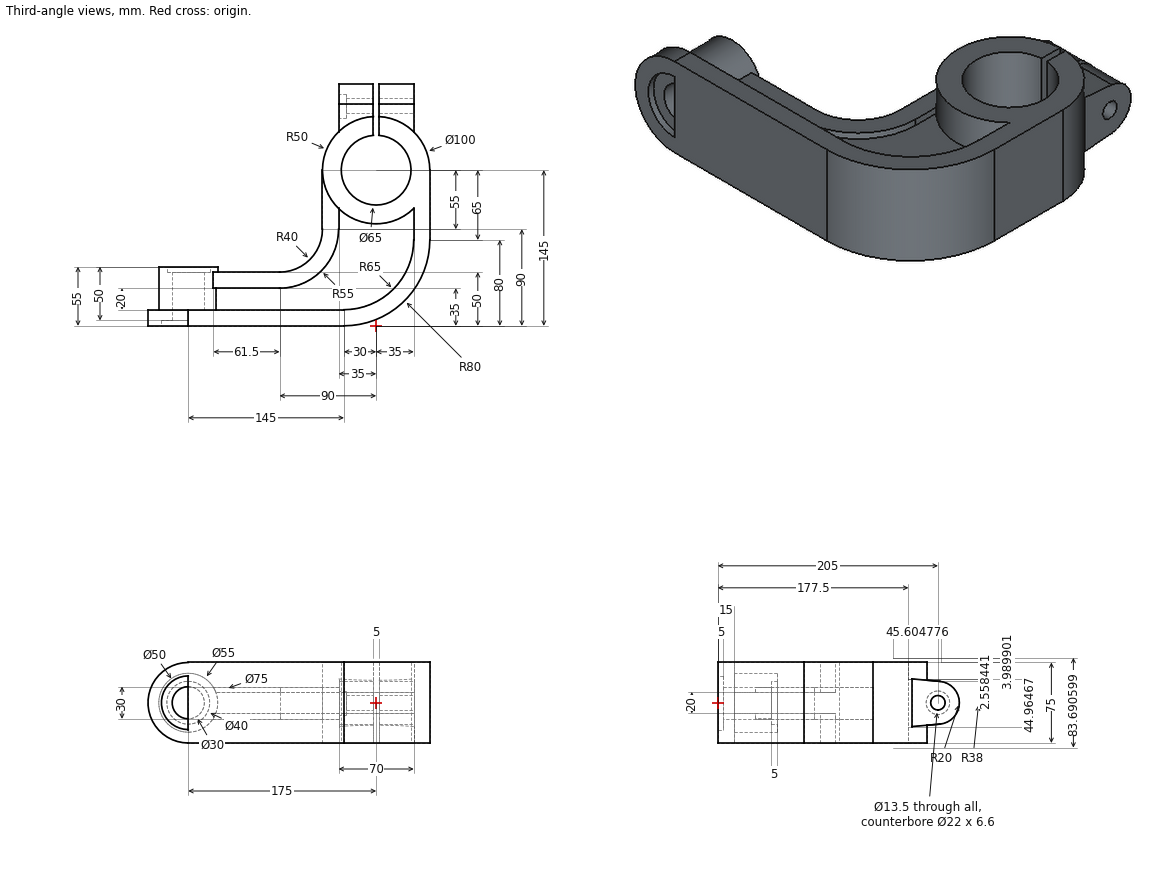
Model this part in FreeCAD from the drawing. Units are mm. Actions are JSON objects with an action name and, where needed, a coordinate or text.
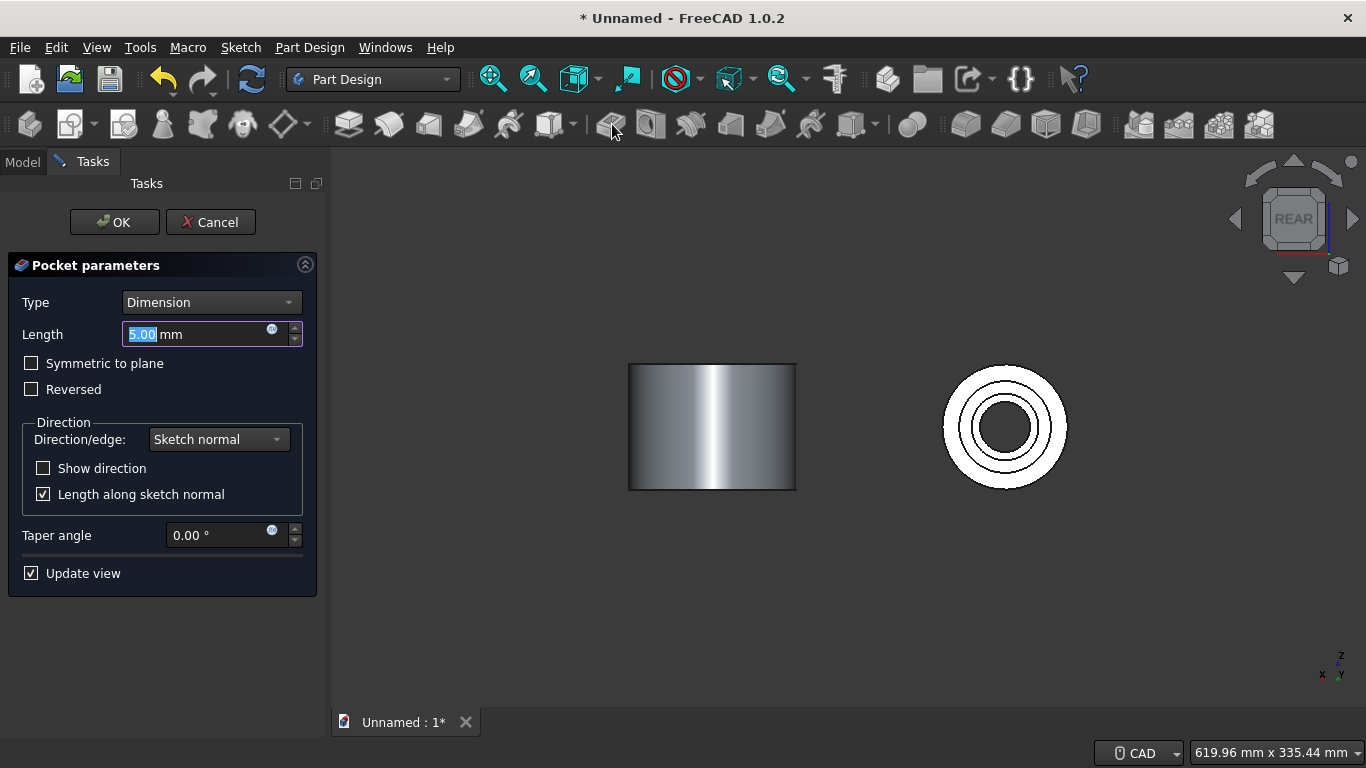
{"action": "type", "text": "5"}
{"action": "key", "text": "Tab"}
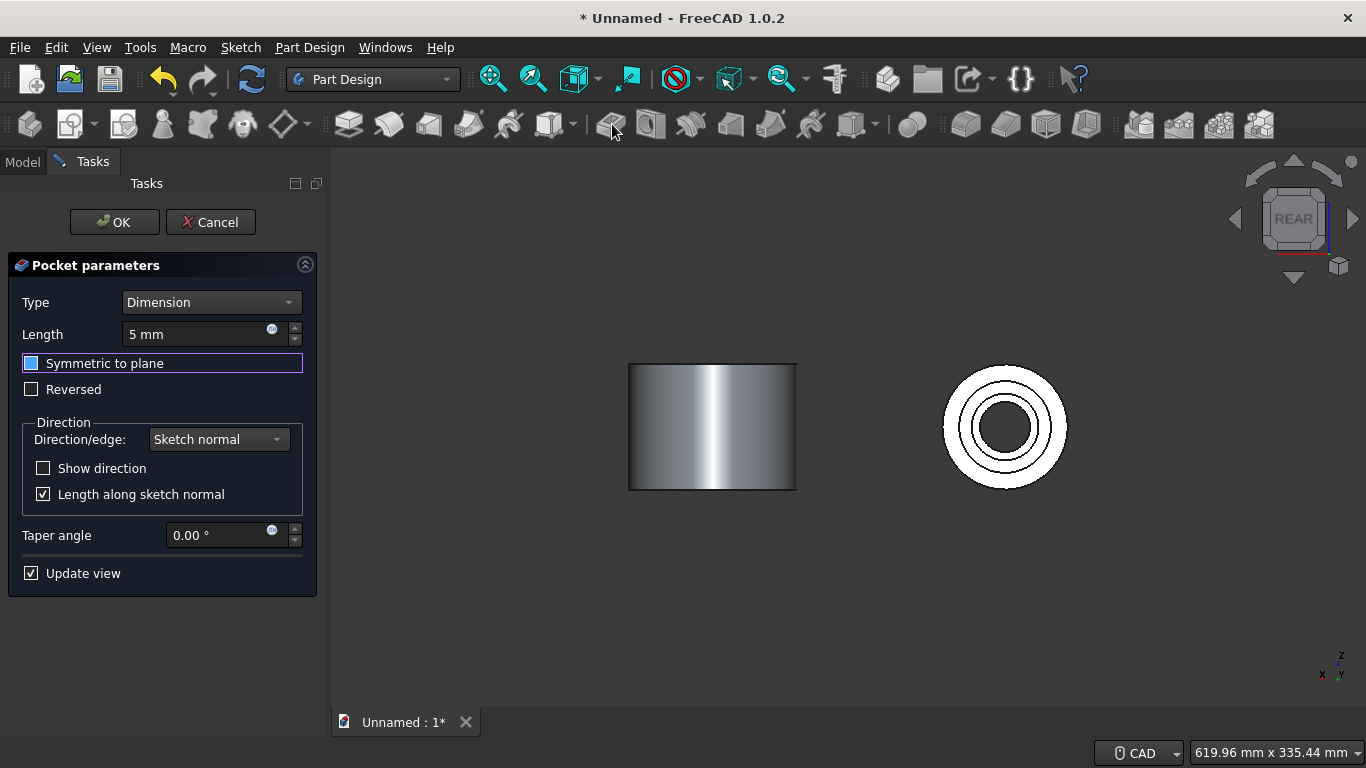
{"action": "left_click", "coordinate": [115, 222]}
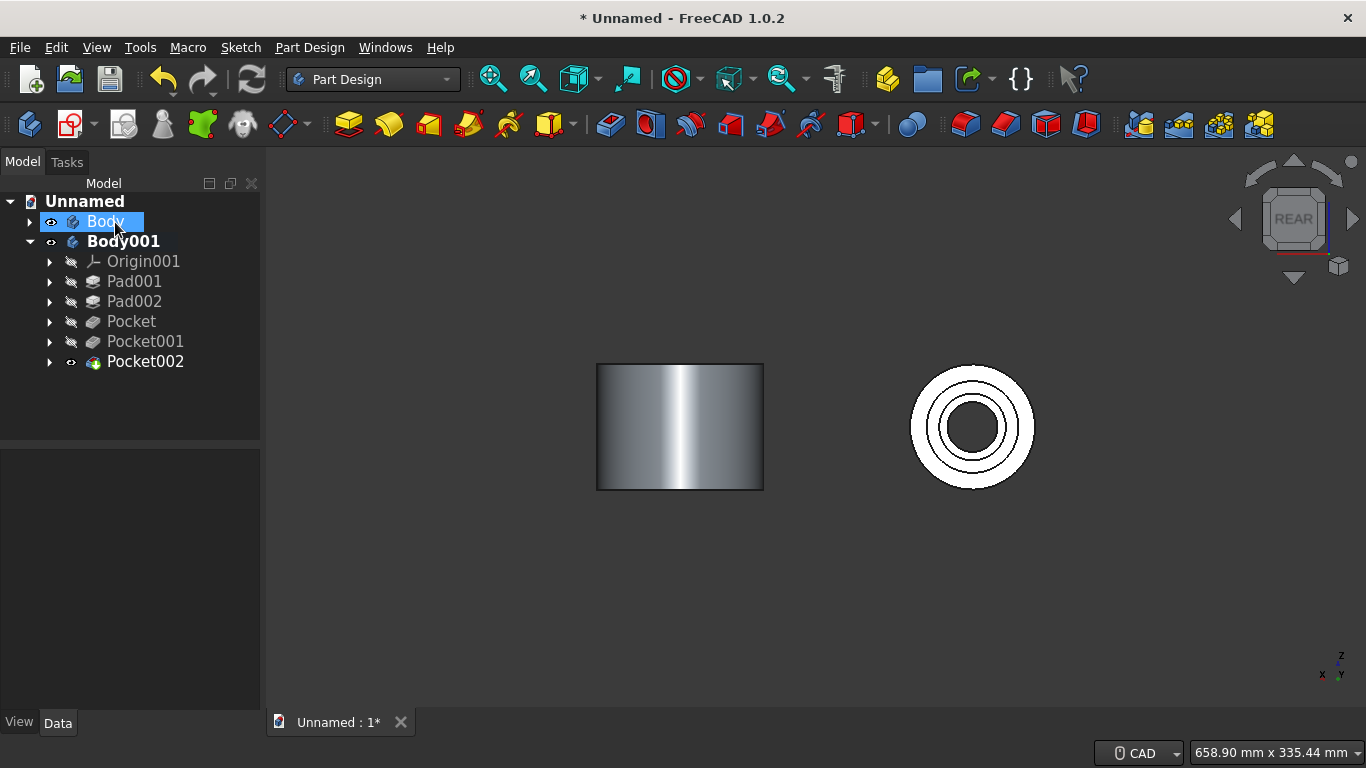
{"action": "key", "text": "v f"}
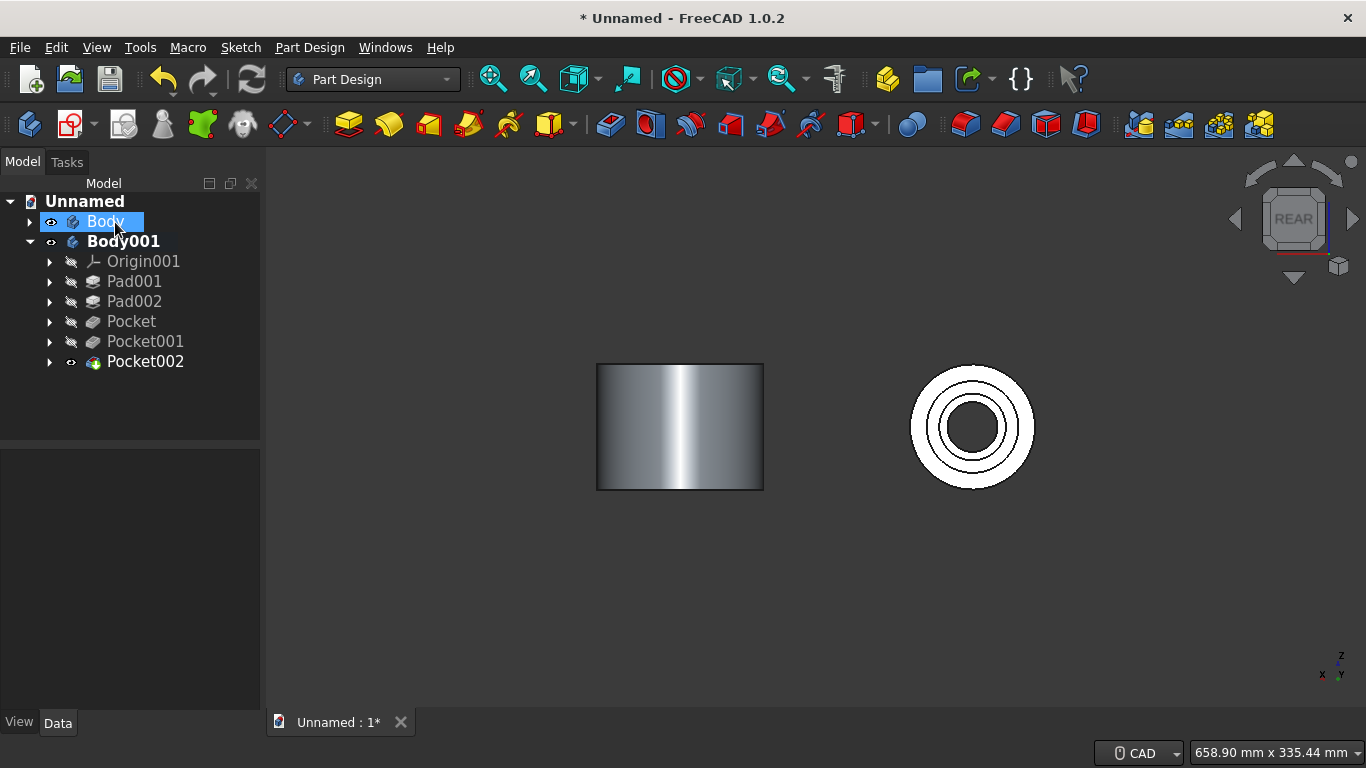
{"action": "double_click", "coordinate": [96, 222]}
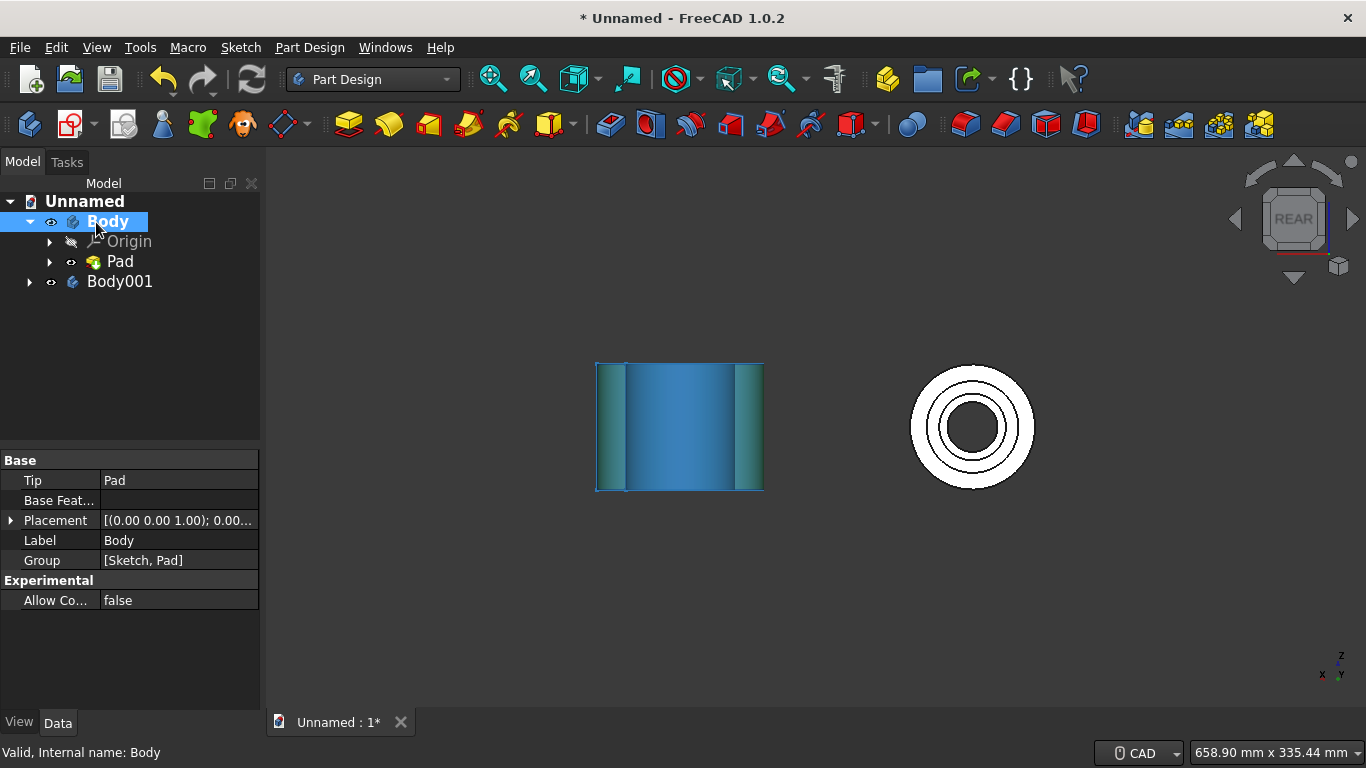
{"action": "left_click", "coordinate": [96, 222]}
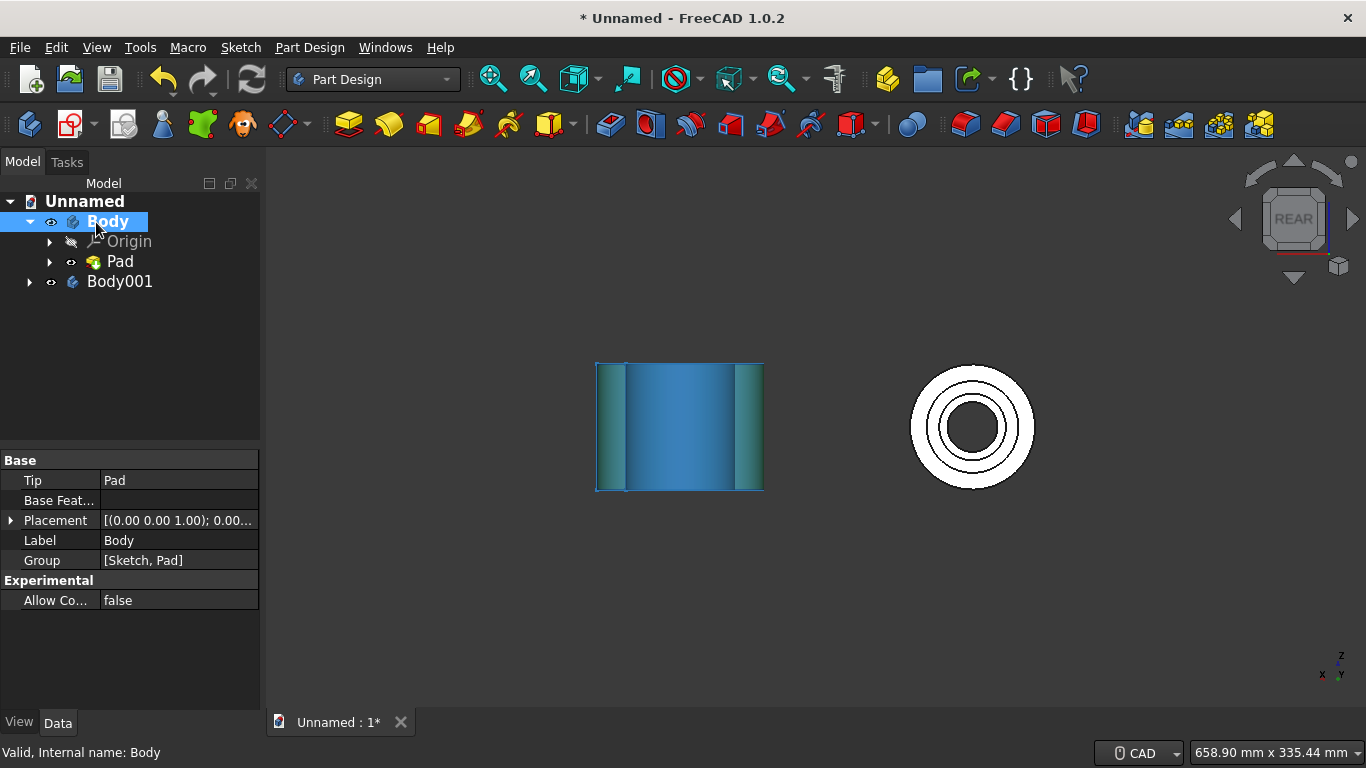
{"action": "left_click", "coordinate": [146, 600]}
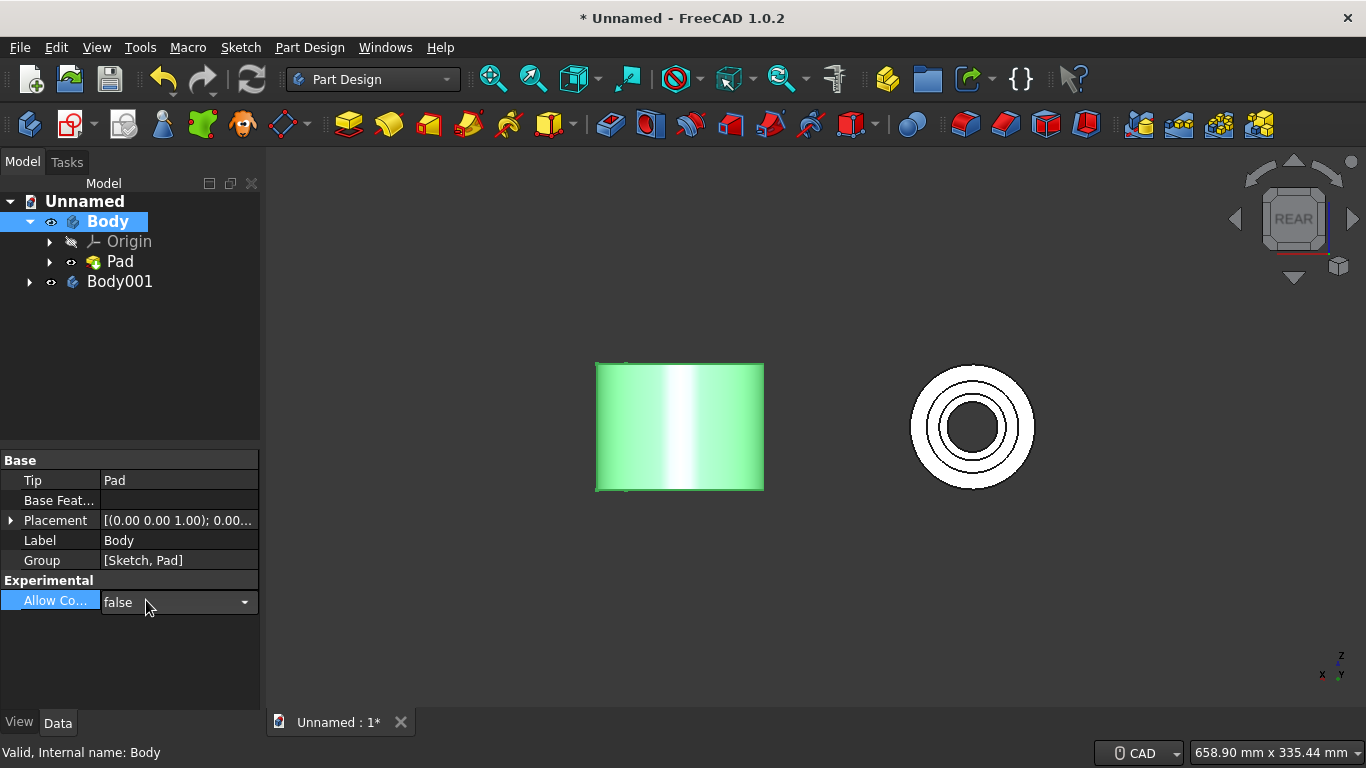
{"action": "left_click", "coordinate": [146, 600]}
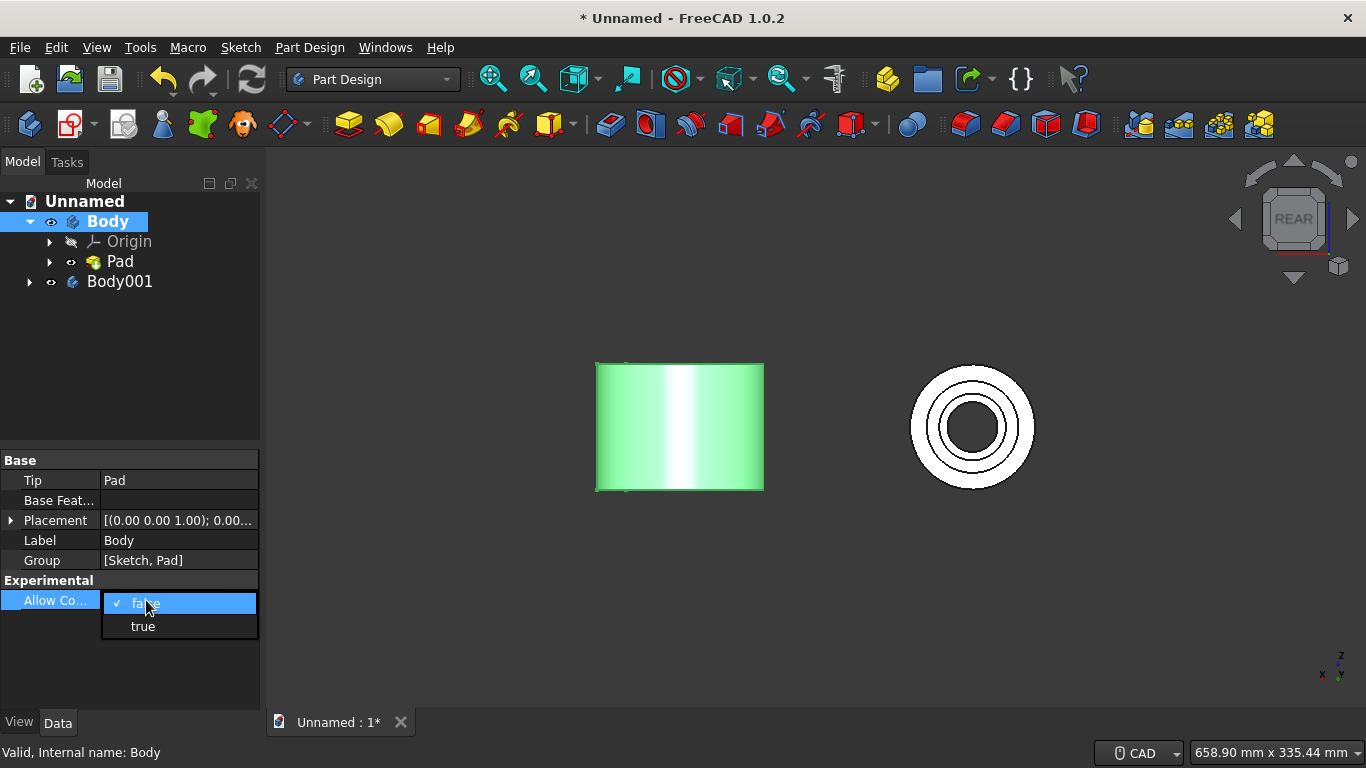
{"action": "left_click", "coordinate": [179, 626]}
{"action": "key", "text": "Return"}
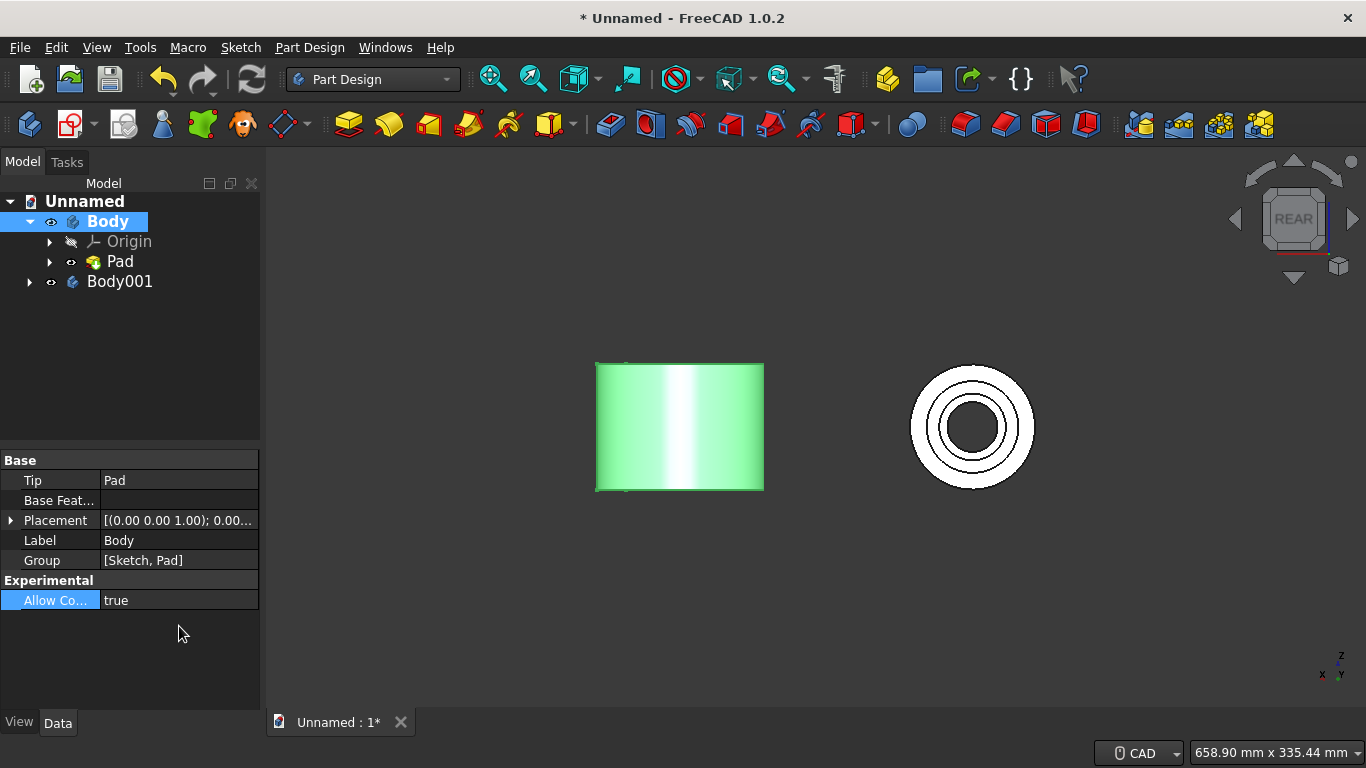
{"action": "left_click", "coordinate": [96, 282]}